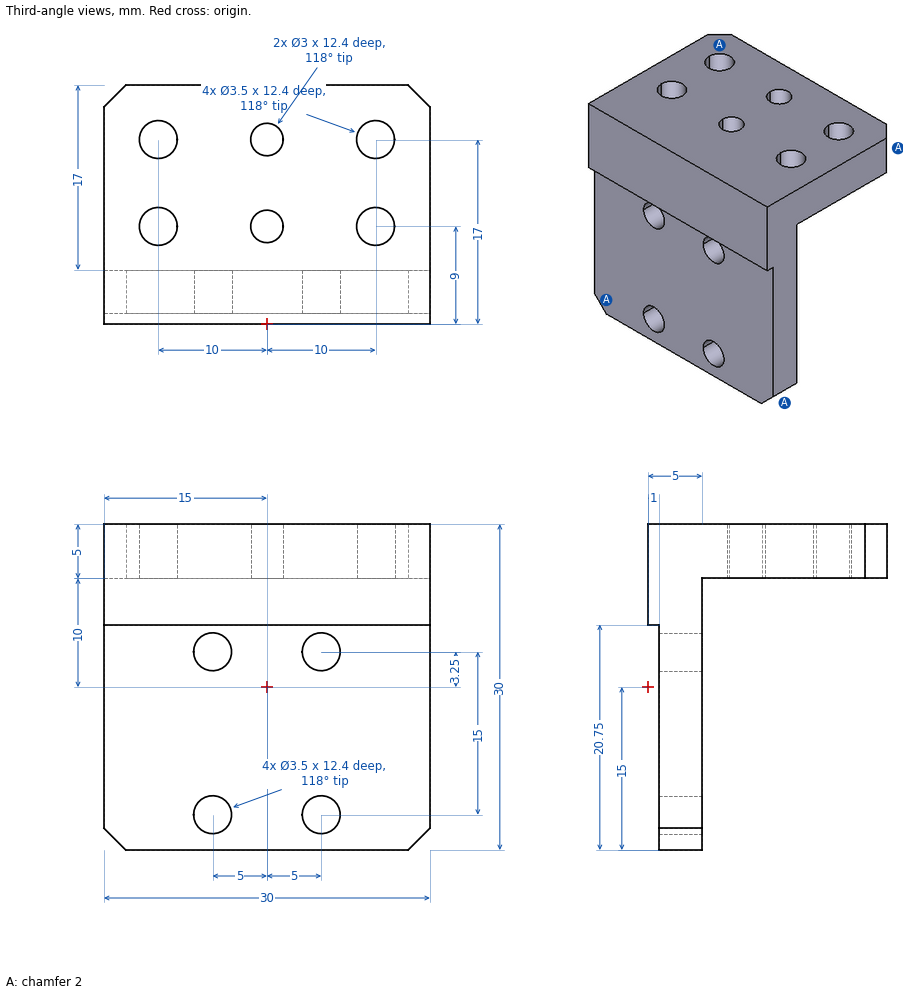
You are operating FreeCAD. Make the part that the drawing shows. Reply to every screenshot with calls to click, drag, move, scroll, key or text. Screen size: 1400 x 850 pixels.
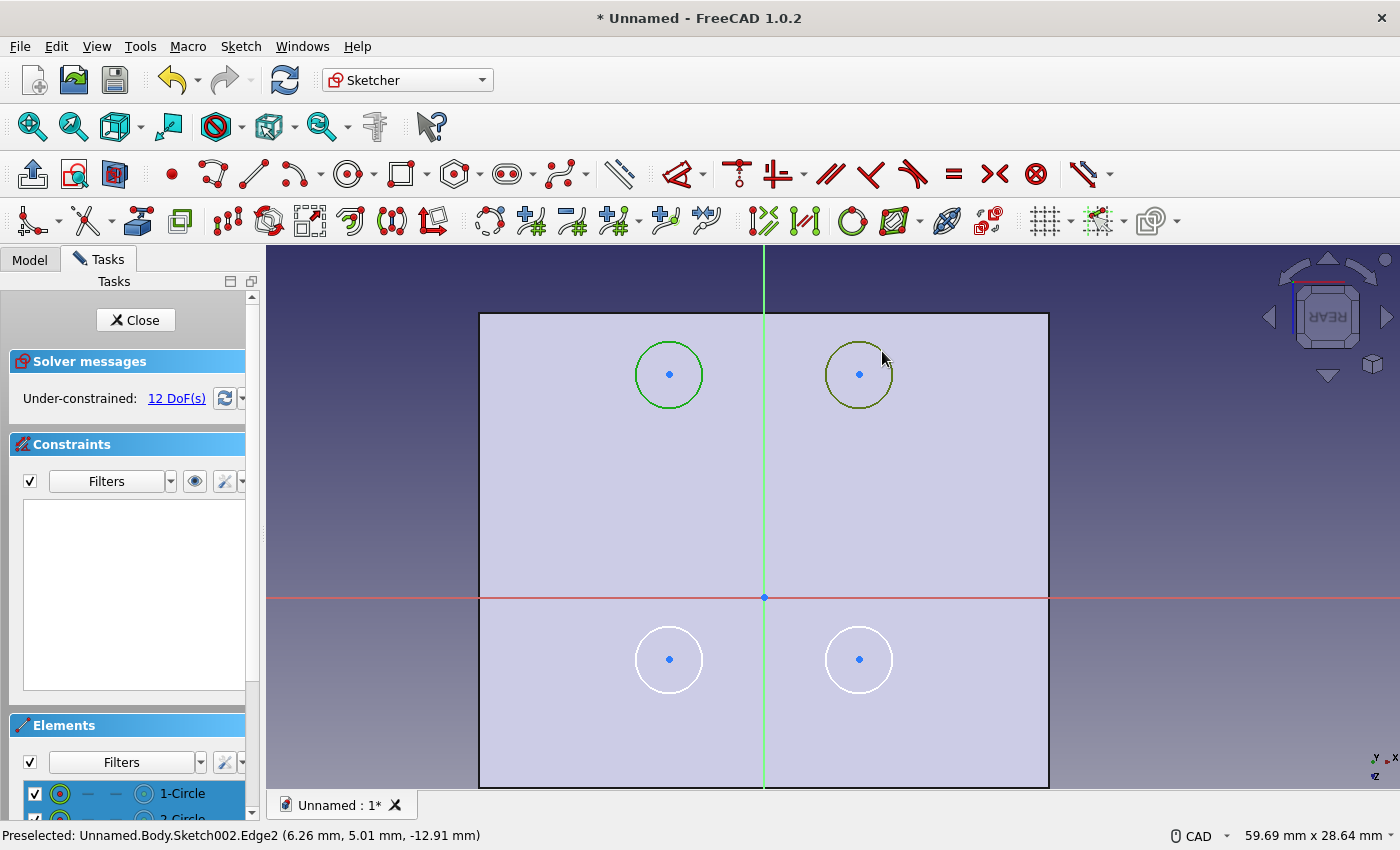
click(882, 636)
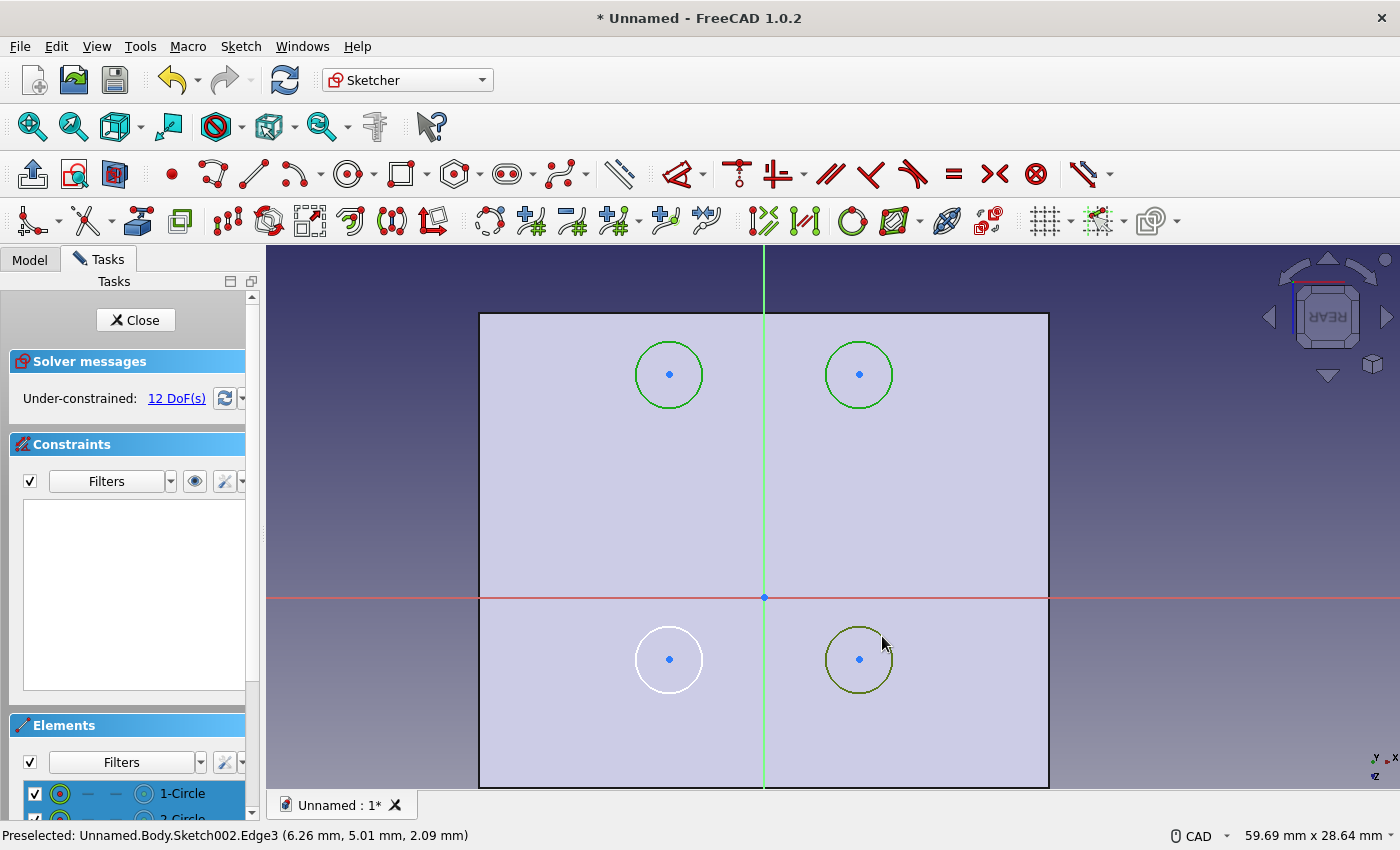
click(692, 636)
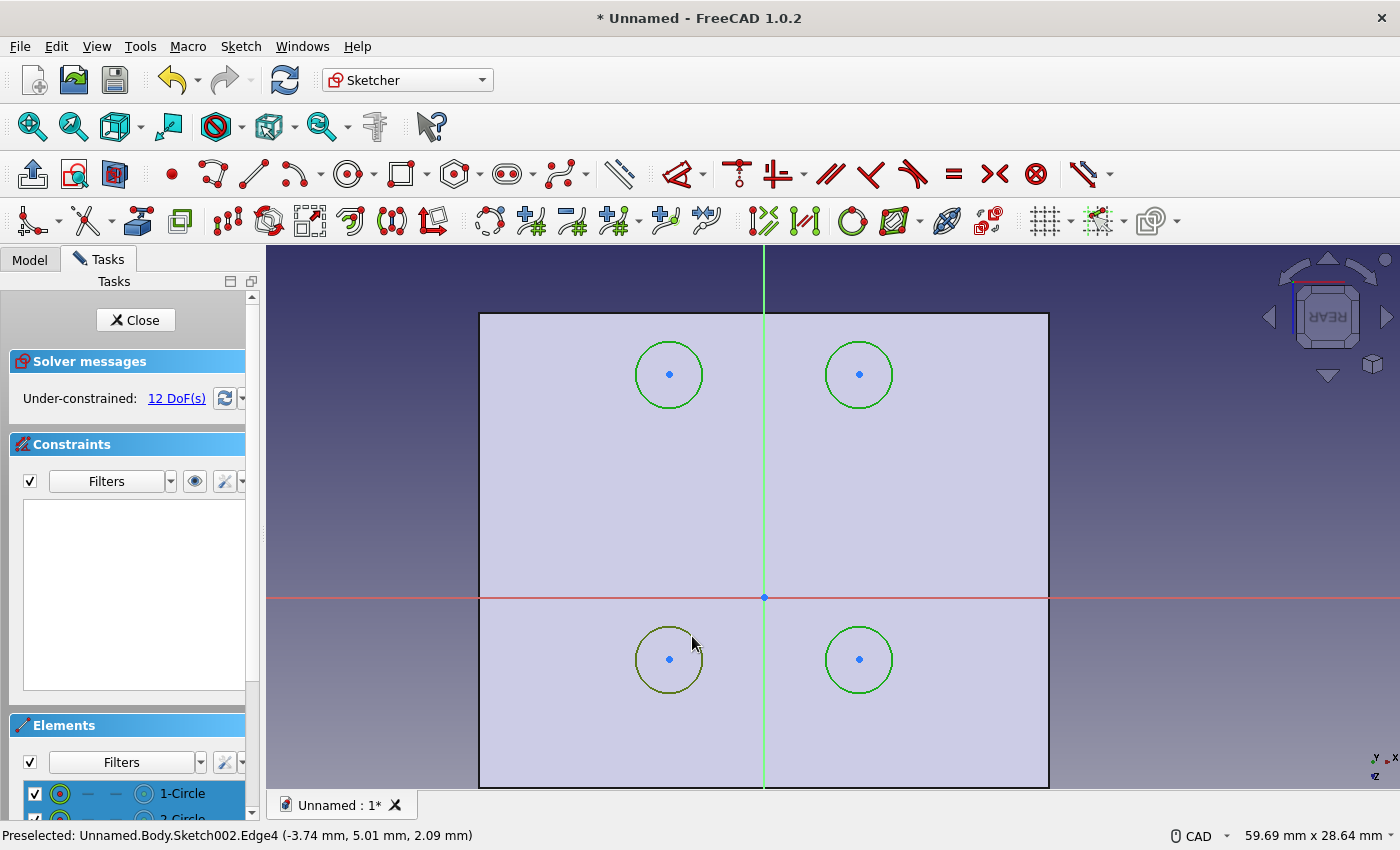
key(e)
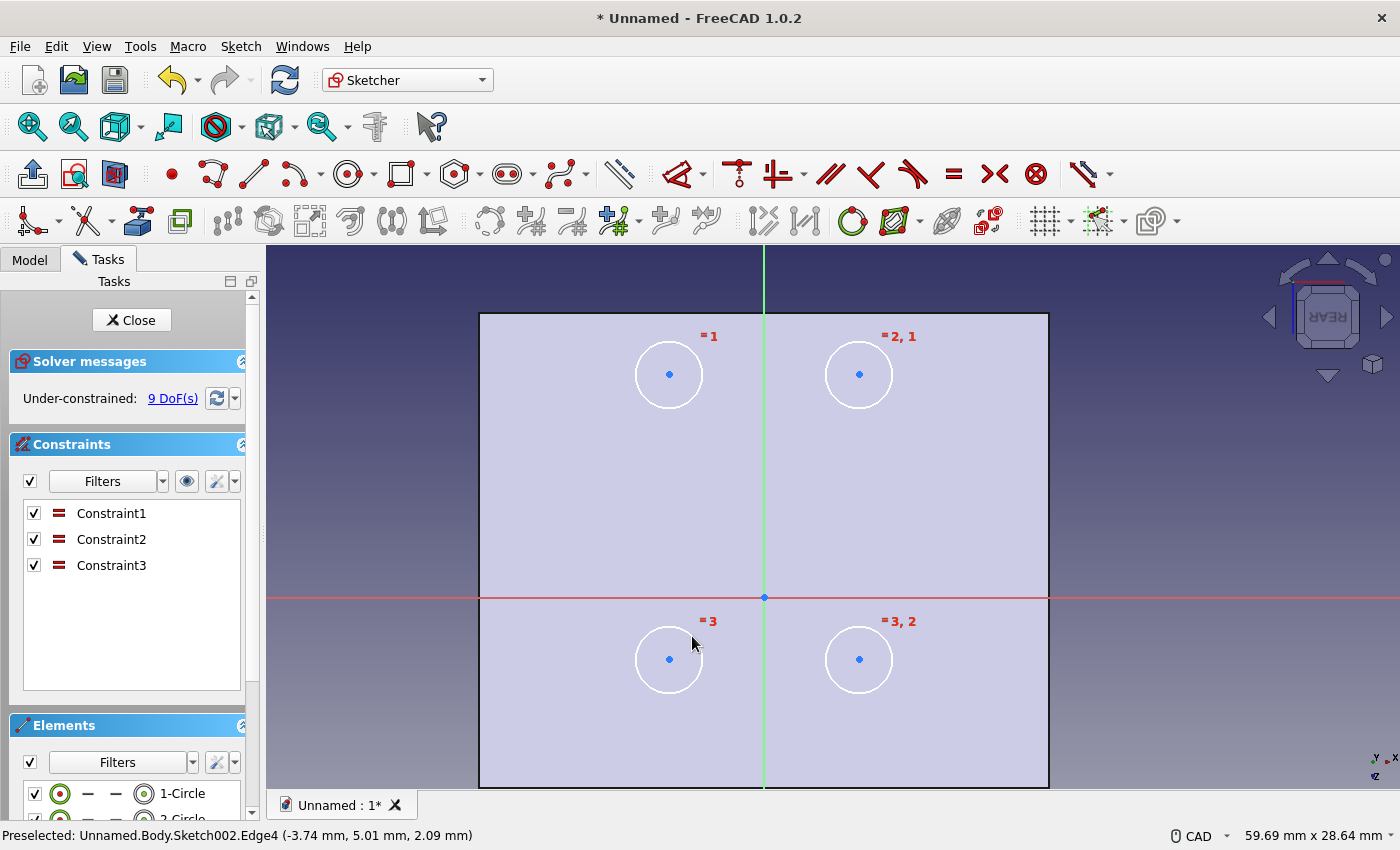
click(669, 375)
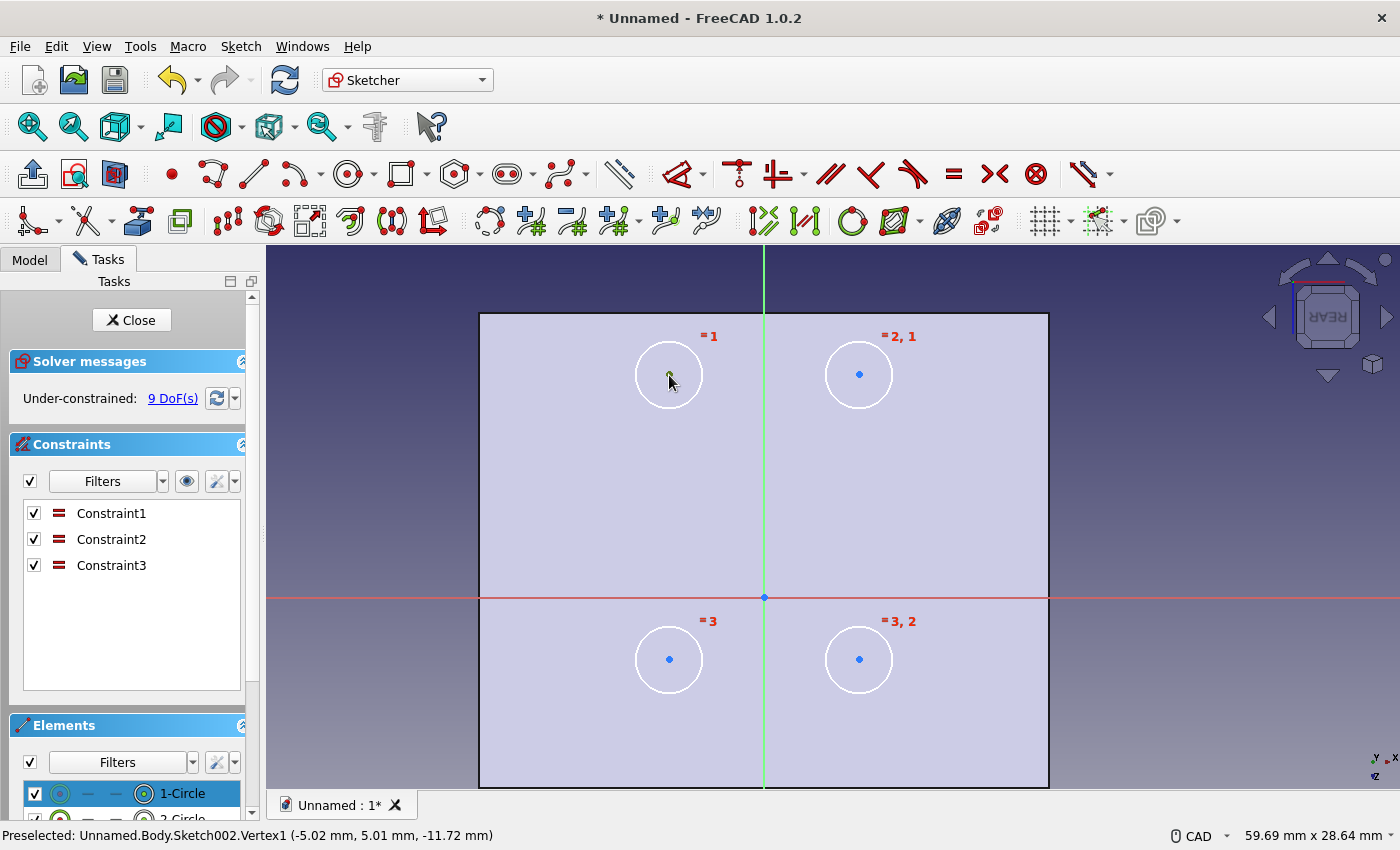
click(859, 375)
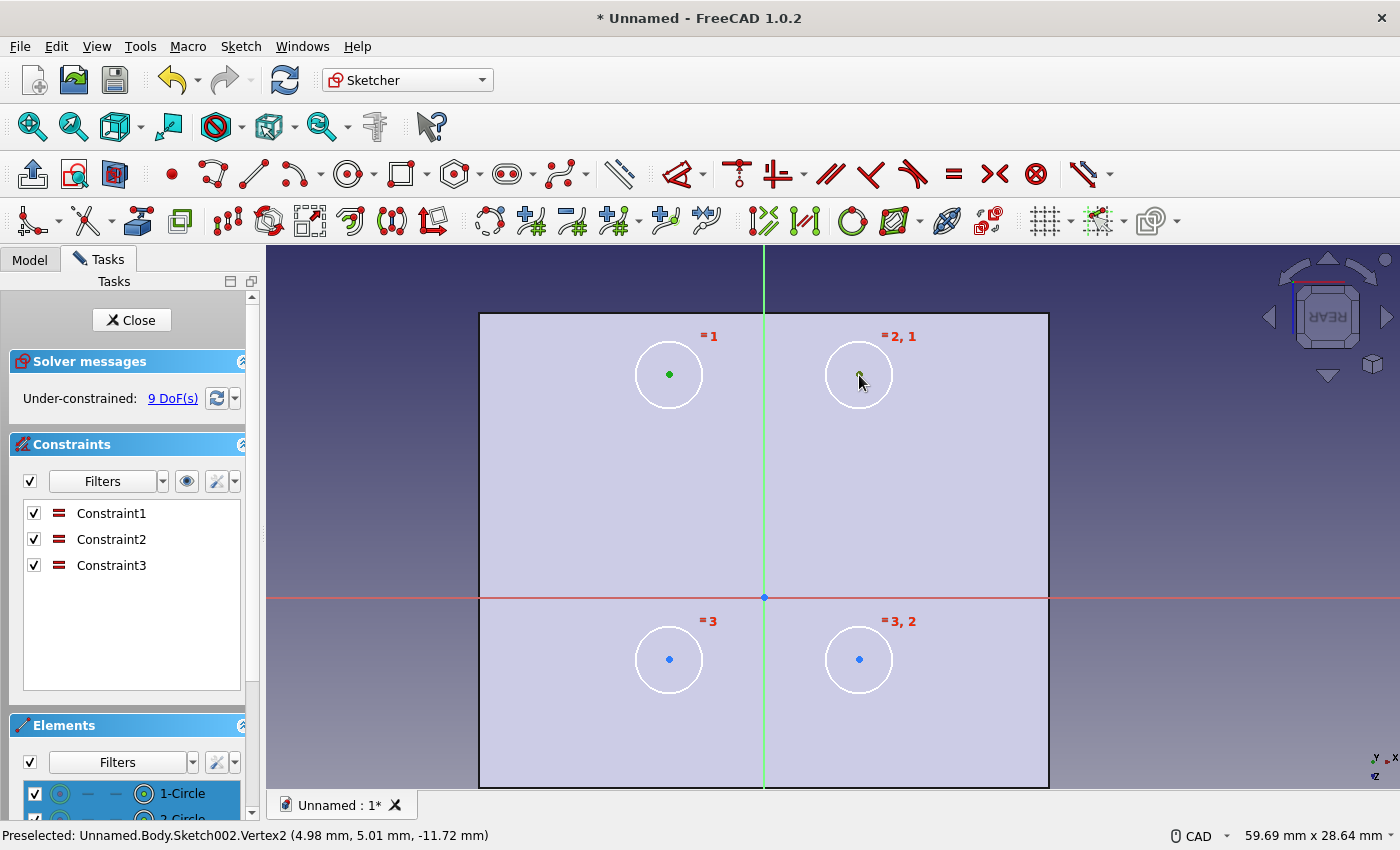
key(h)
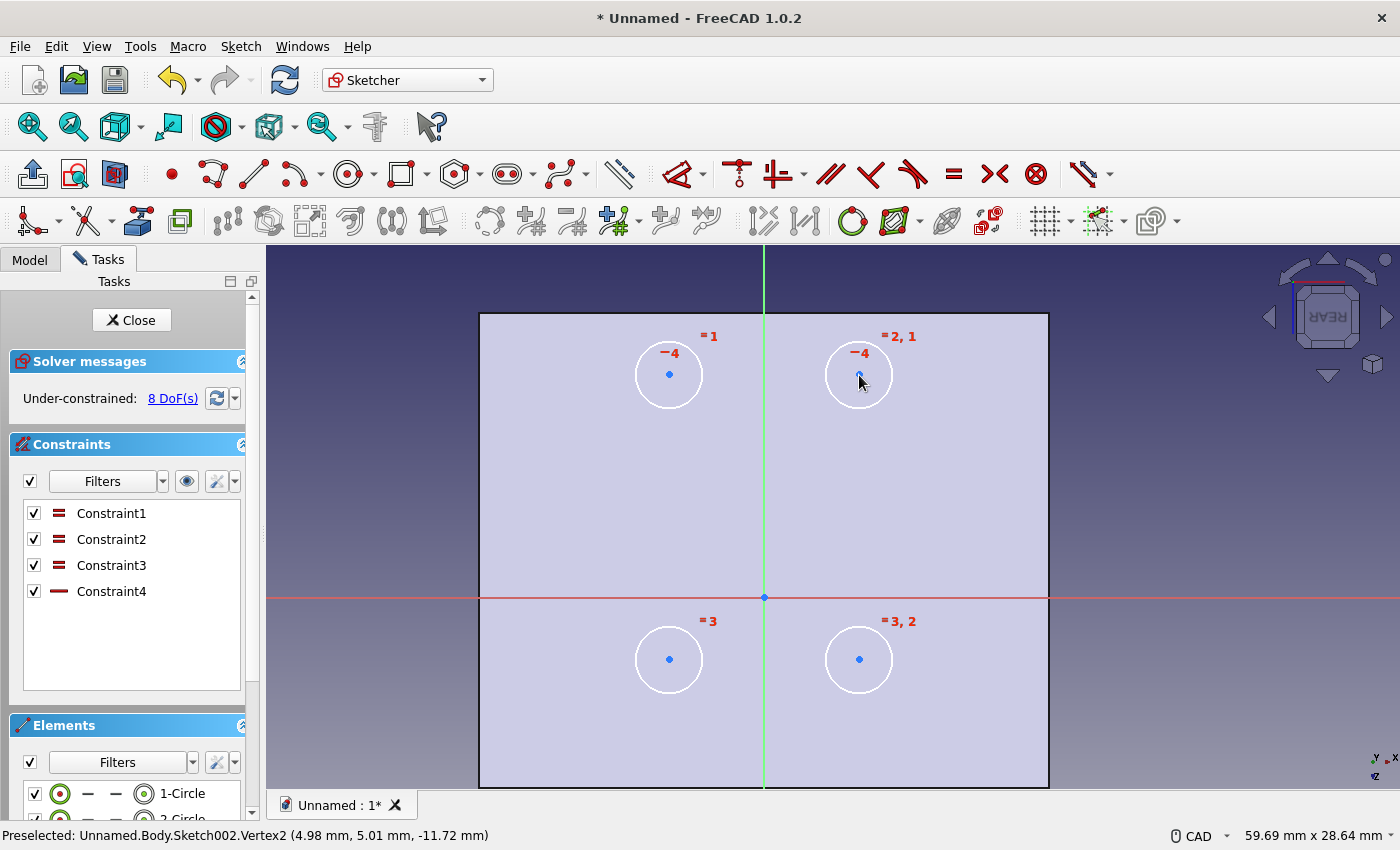
click(859, 375)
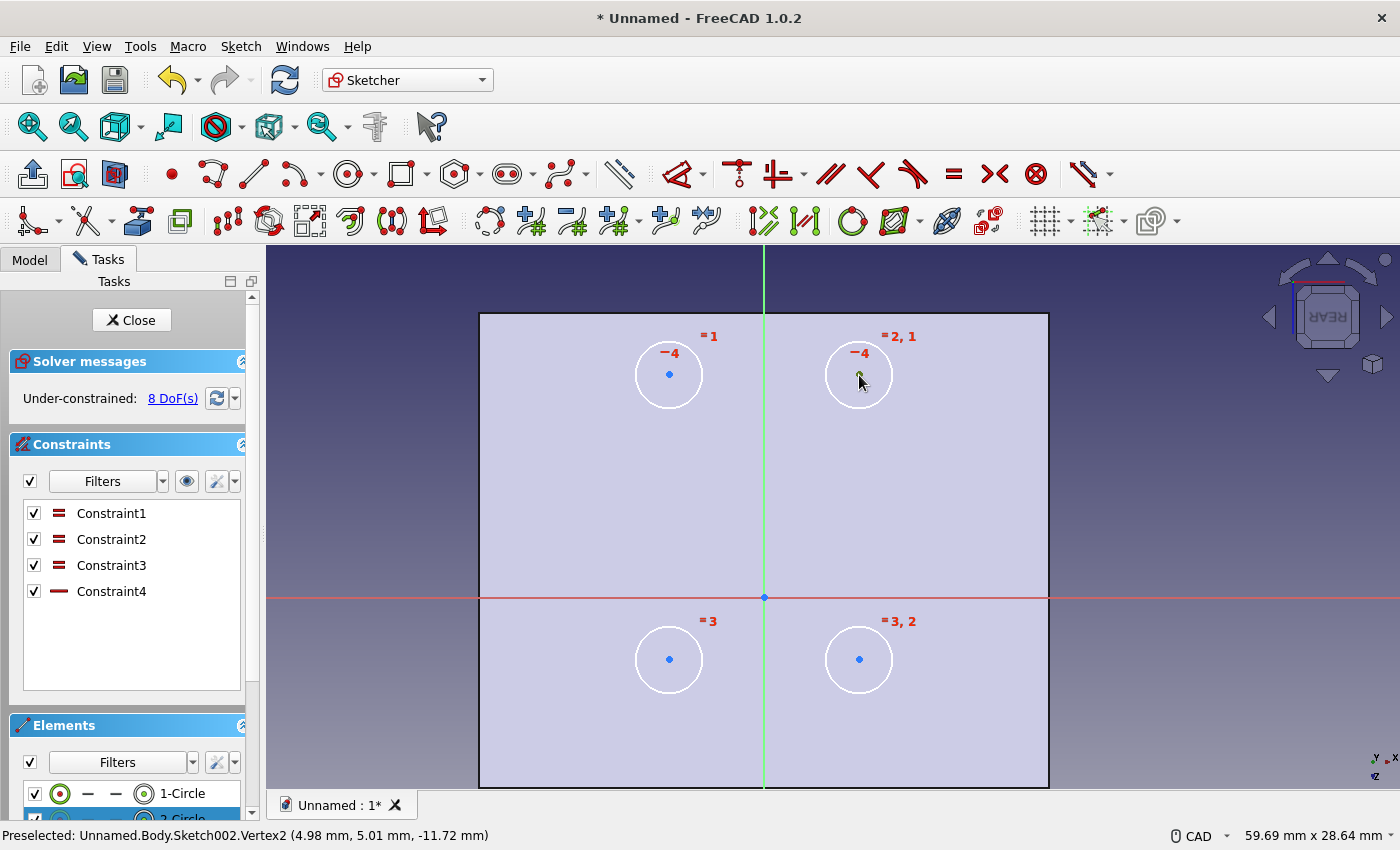
click(859, 660)